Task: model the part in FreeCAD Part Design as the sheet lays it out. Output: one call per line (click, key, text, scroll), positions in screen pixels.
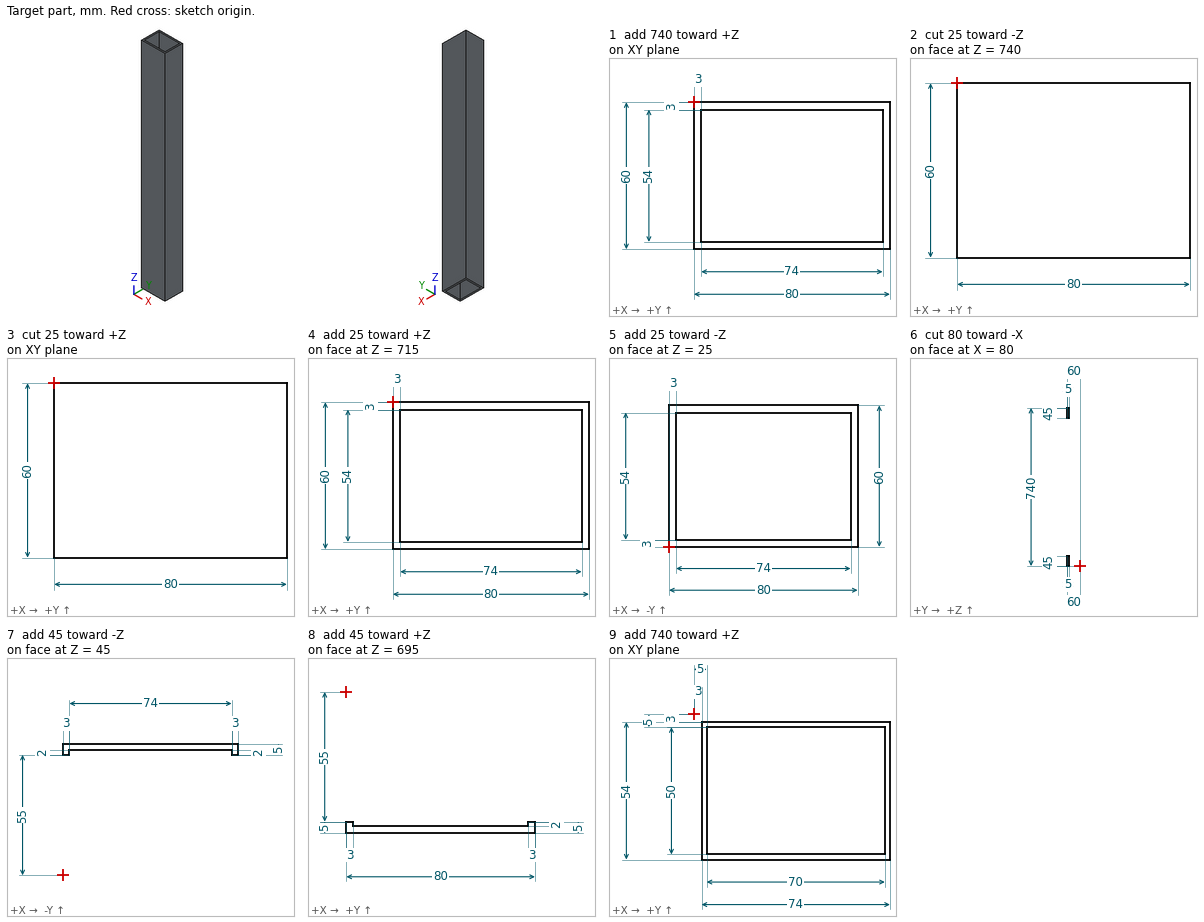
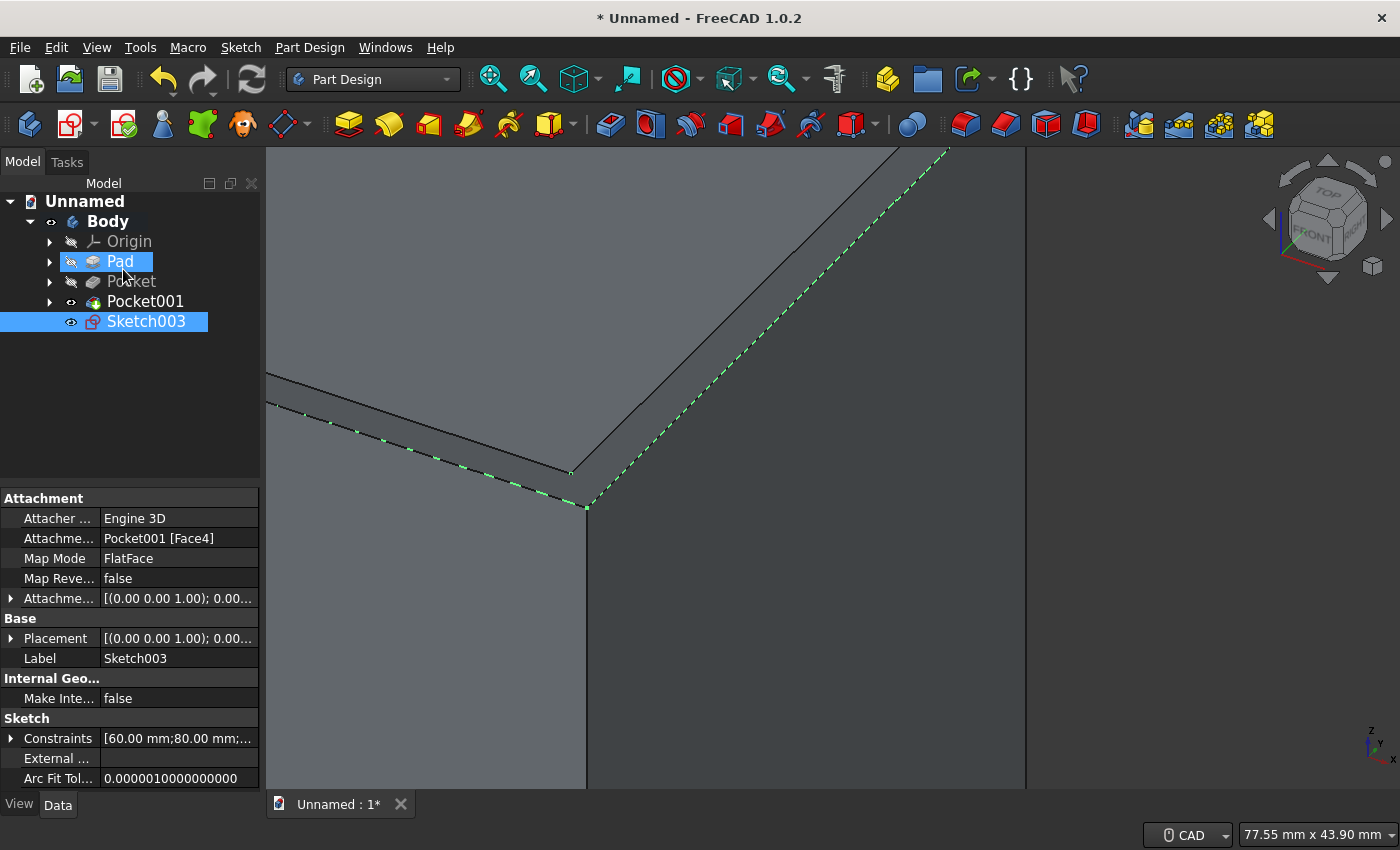
click(350, 124)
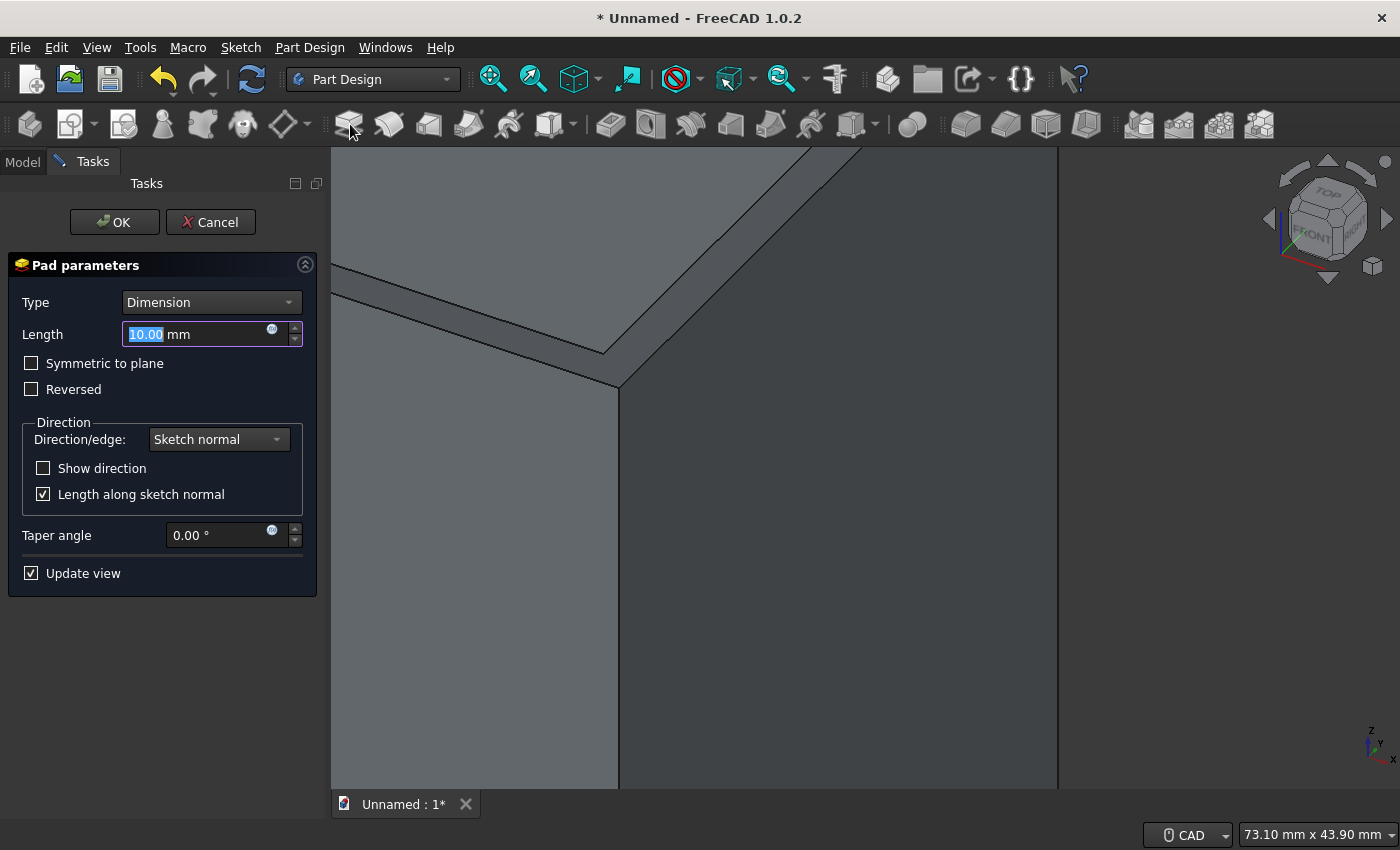
text(25)
key(Tab)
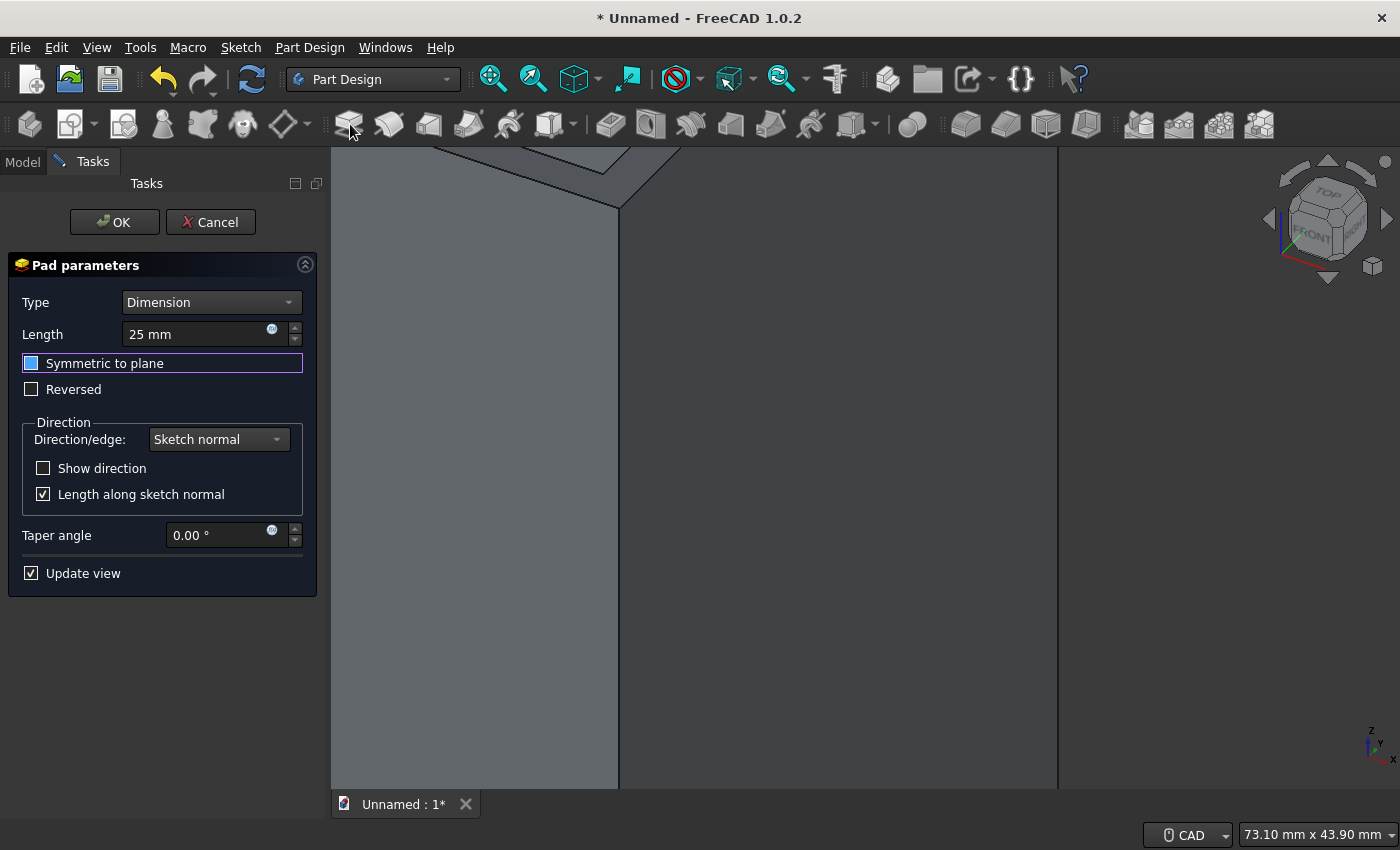
click(115, 222)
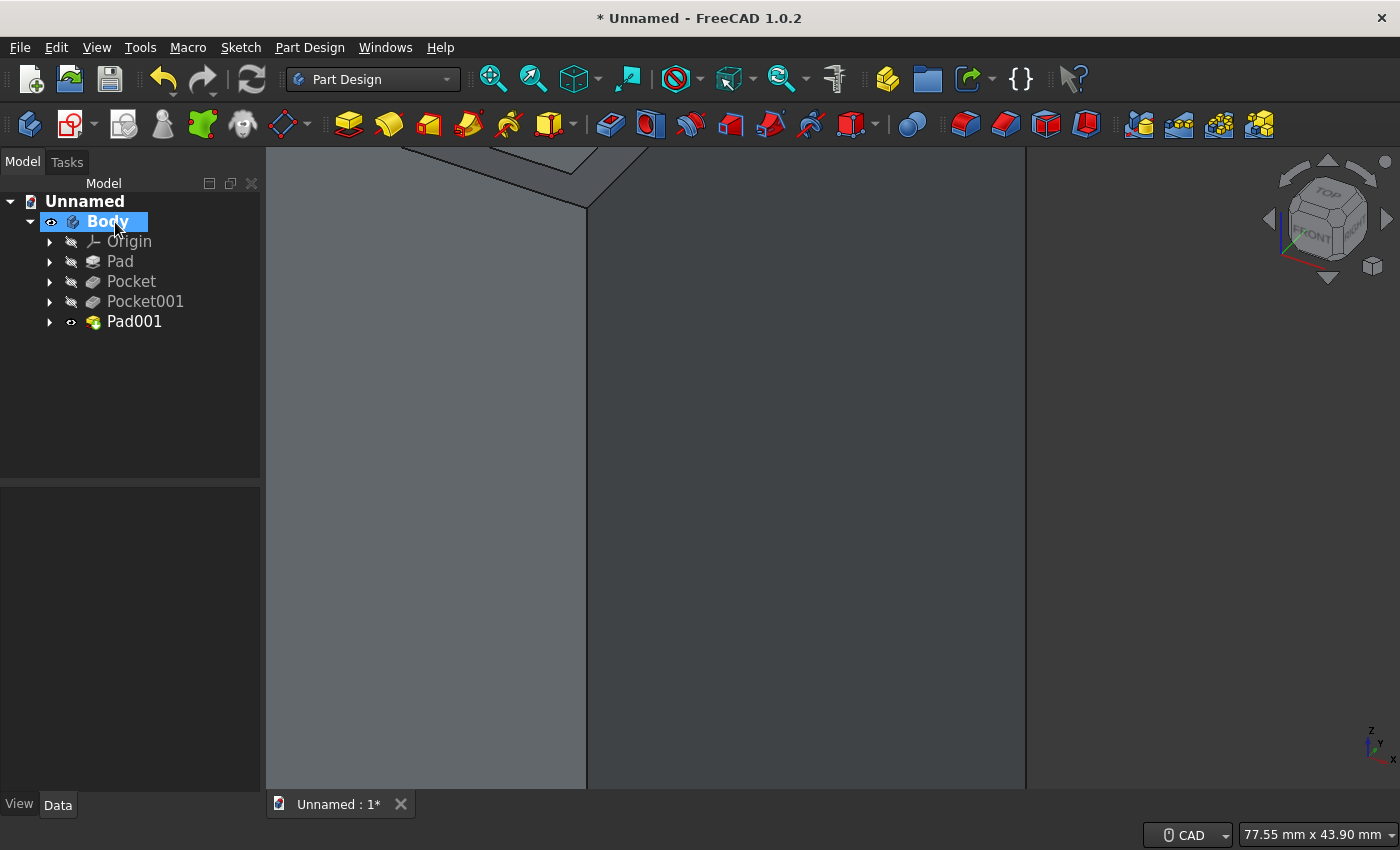
click(494, 80)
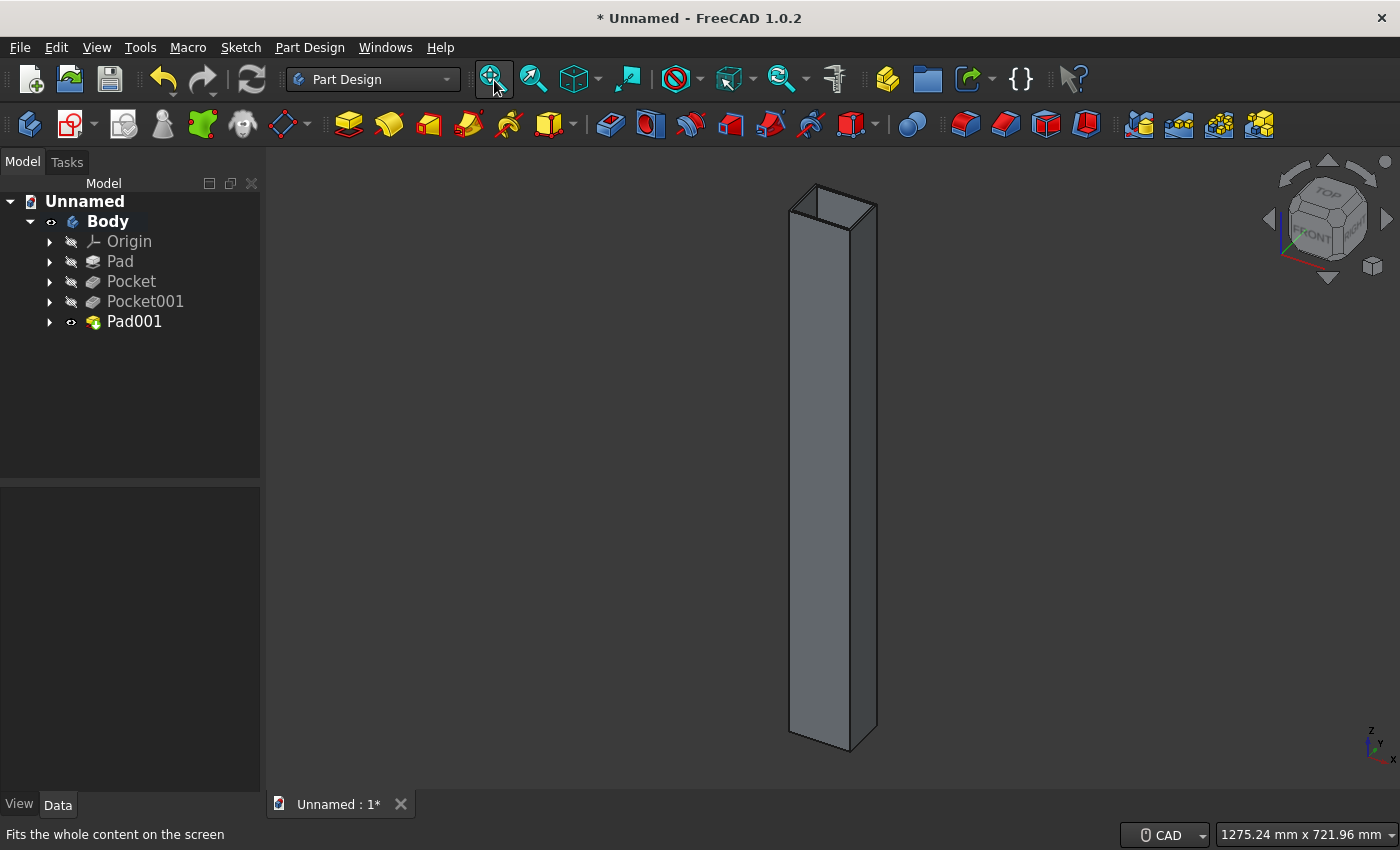
key(5)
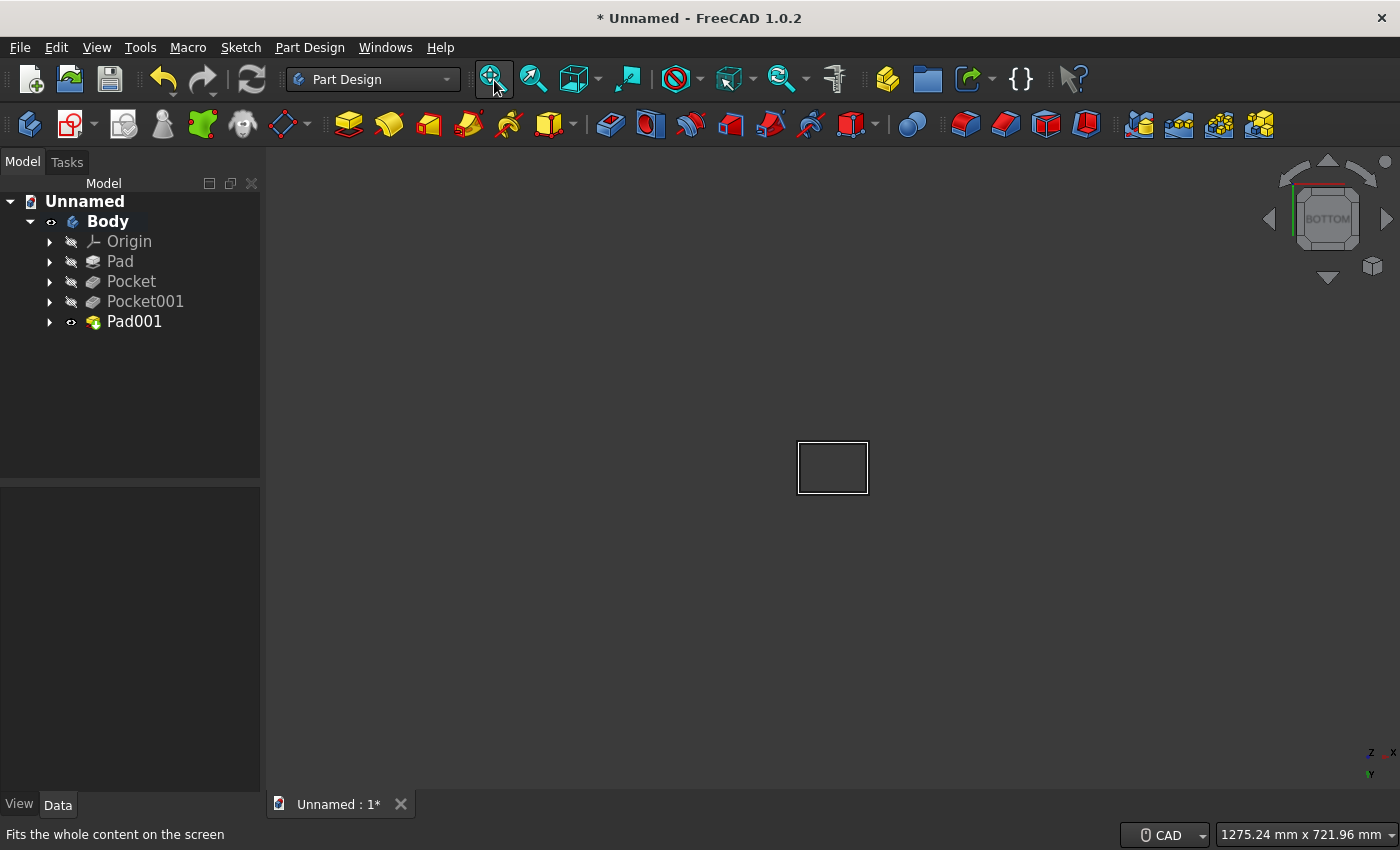
key(v)
key(f)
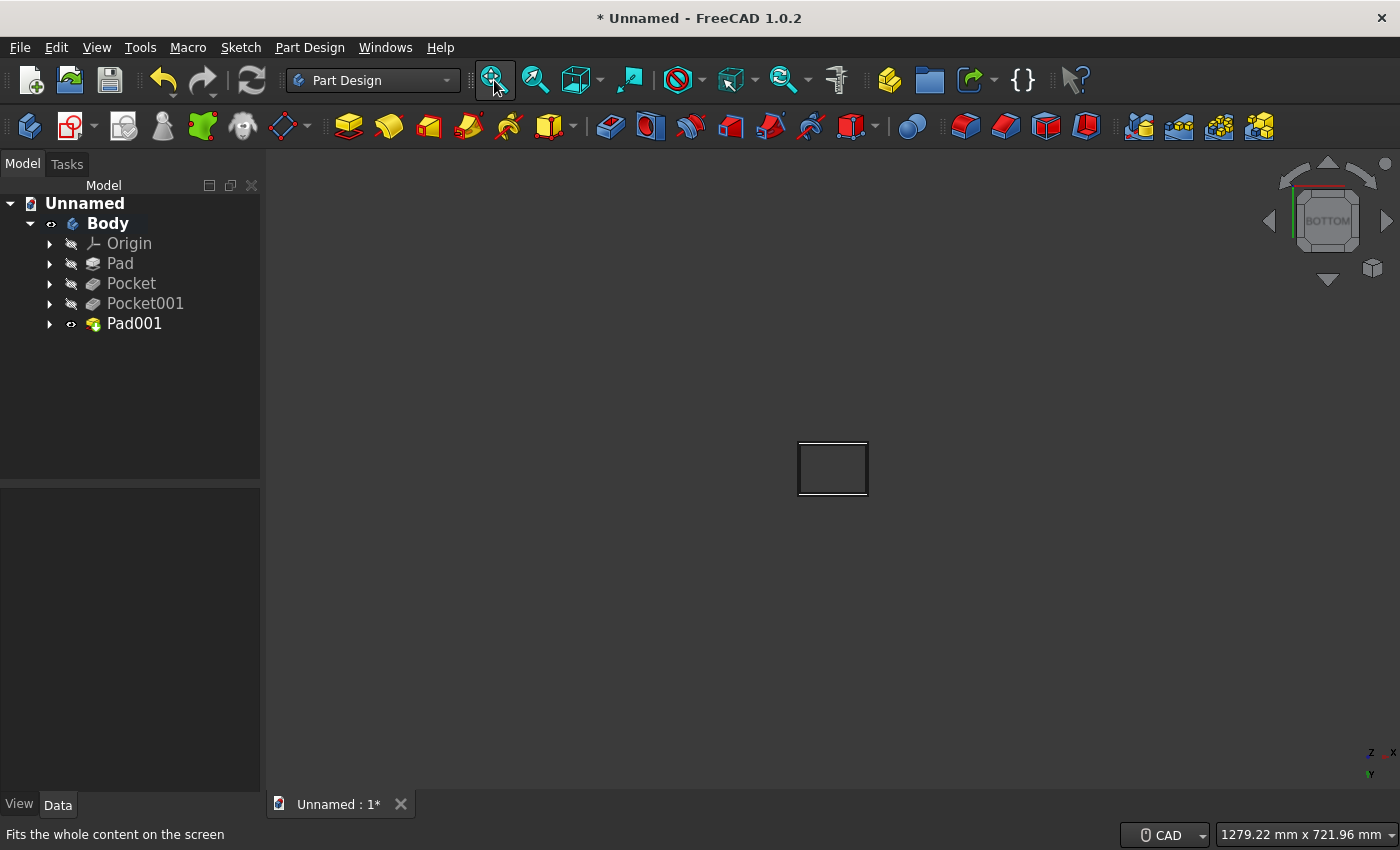
scroll(868, 476, up, 14)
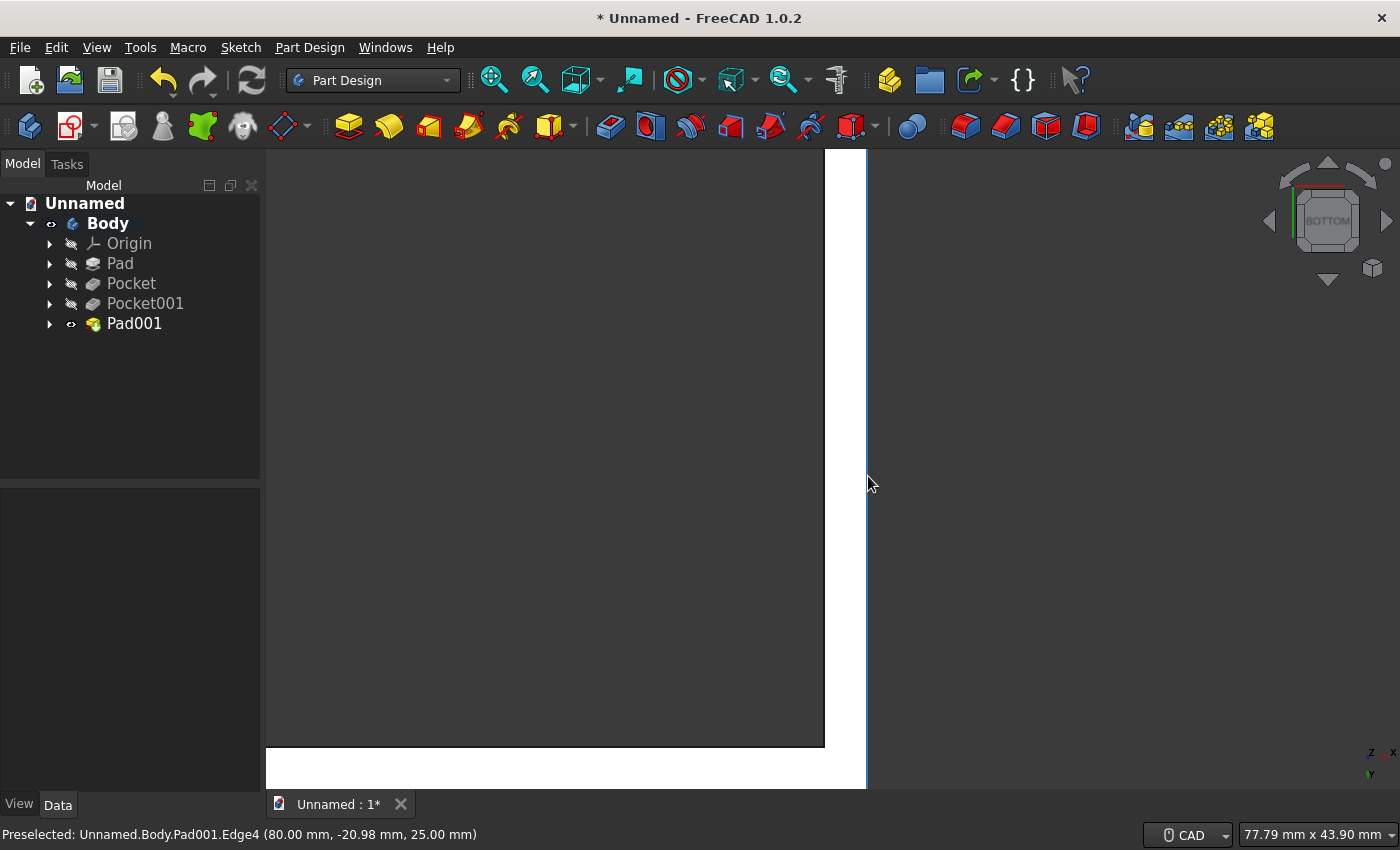
click(853, 483)